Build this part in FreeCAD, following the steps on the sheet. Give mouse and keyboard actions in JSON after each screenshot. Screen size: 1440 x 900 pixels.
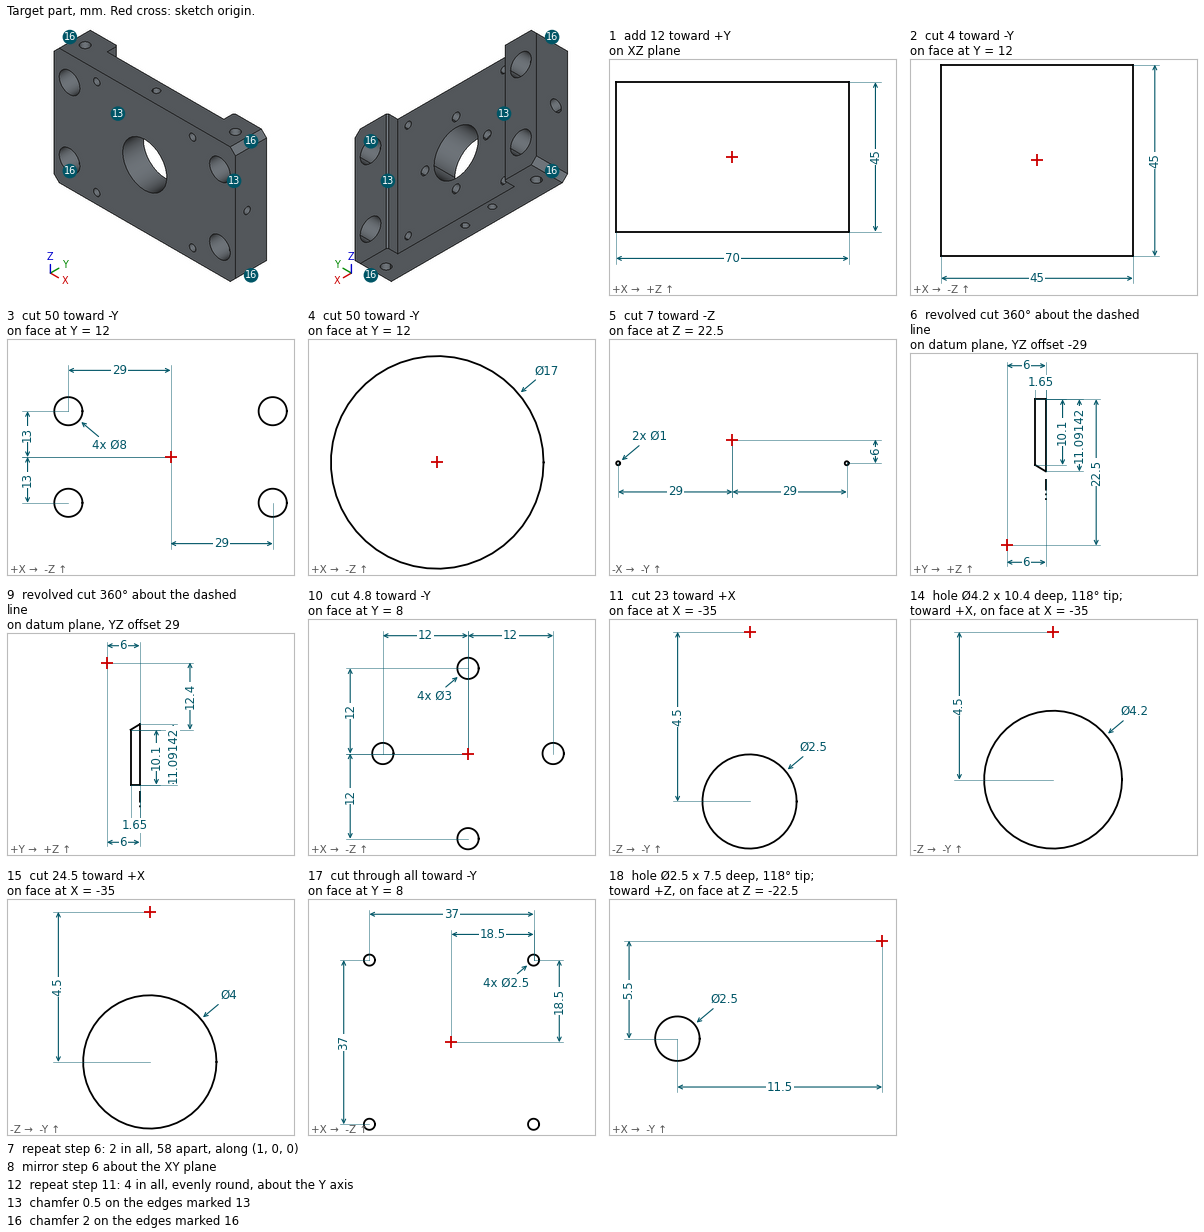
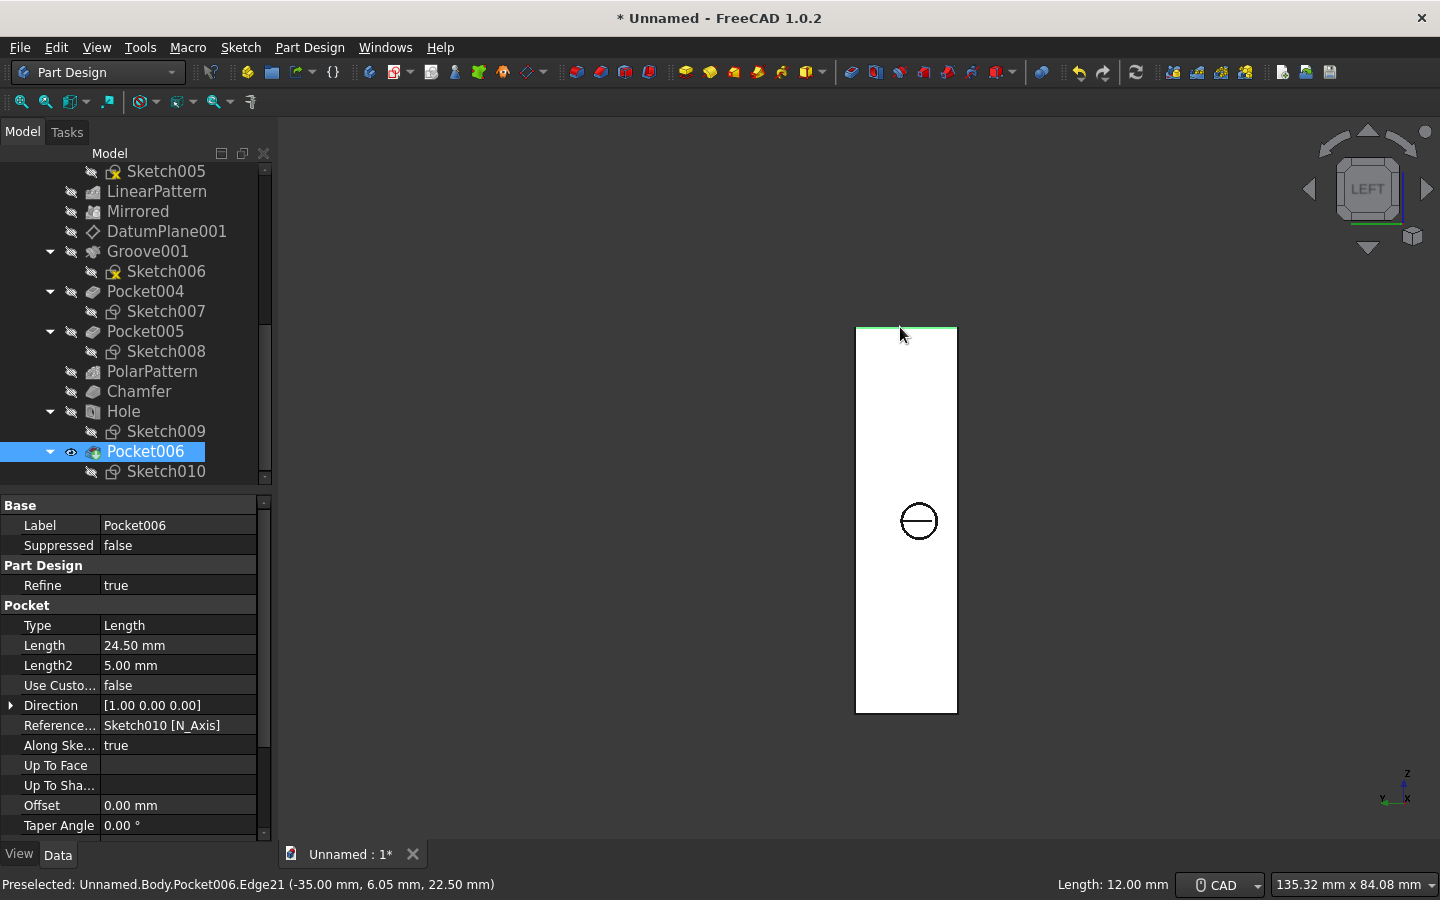
{"action": "left_click", "coordinate": [906, 713], "text": "ctrl"}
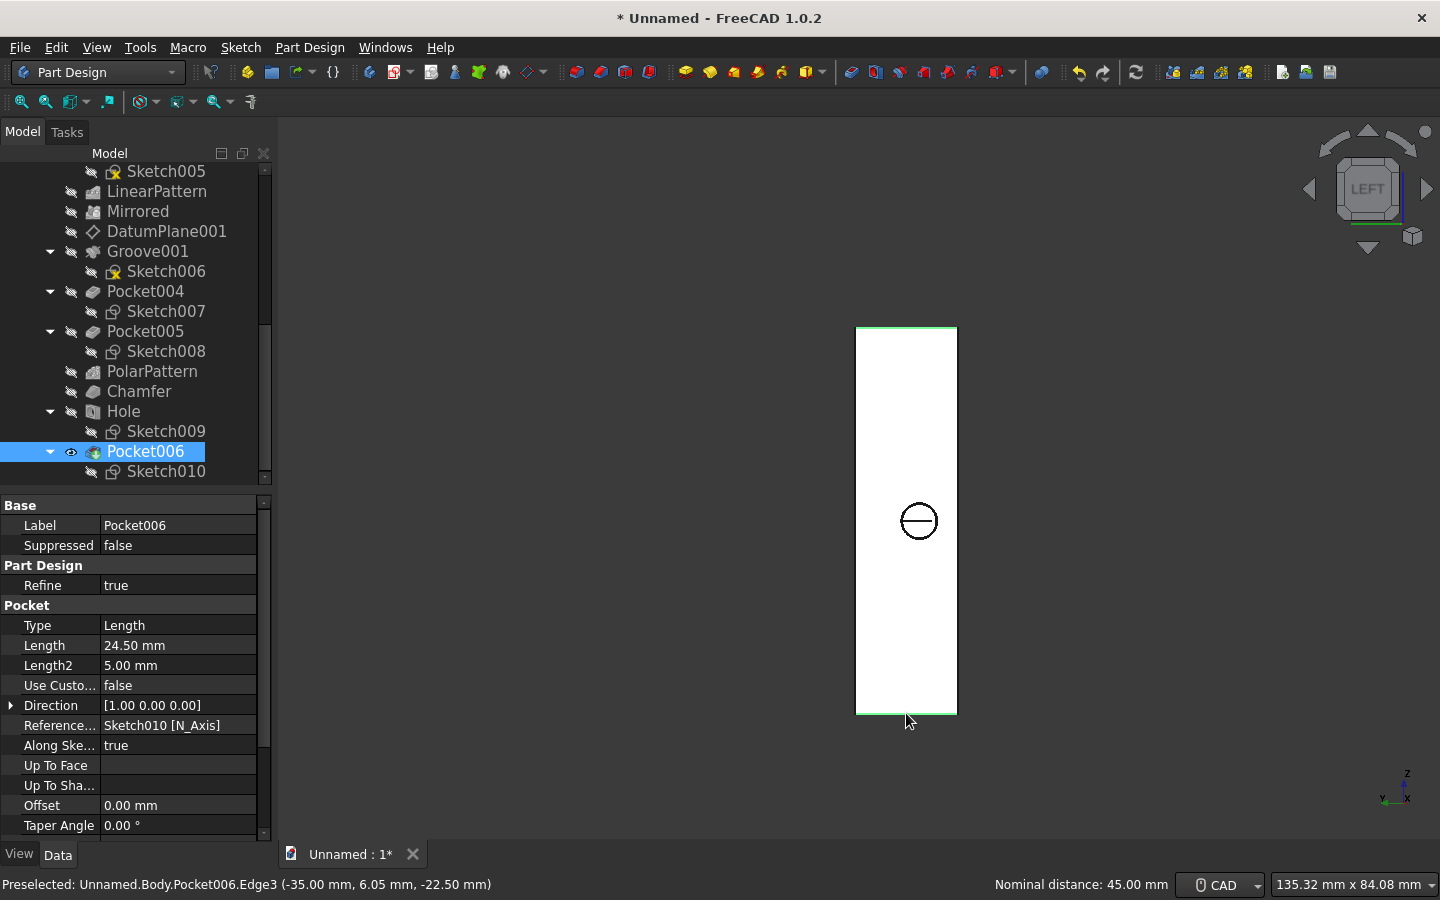
{"action": "key", "text": "0"}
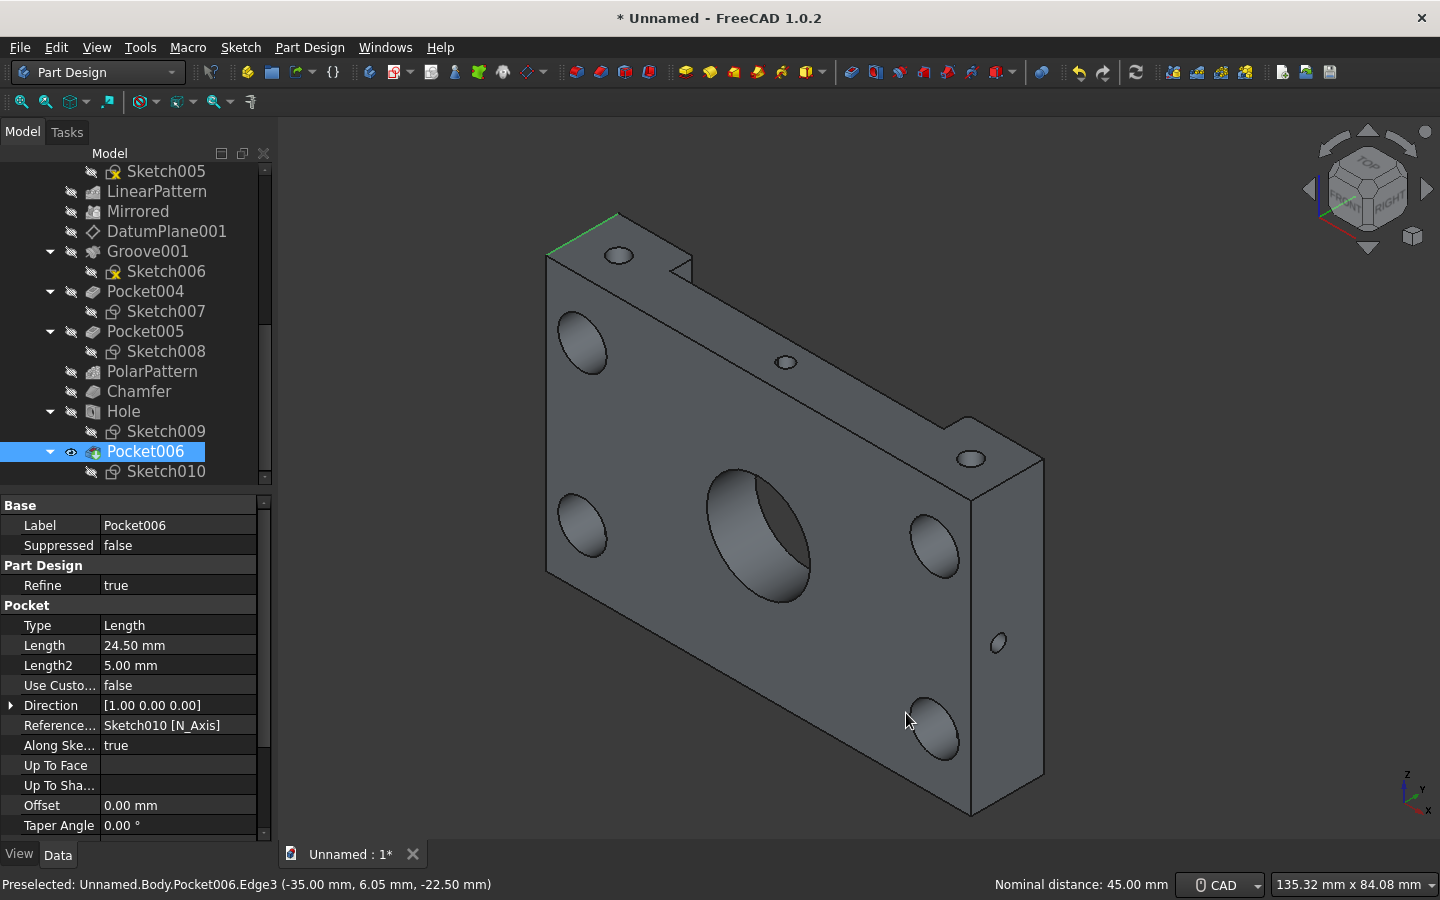
{"action": "left_click", "coordinate": [1007, 479], "text": "ctrl"}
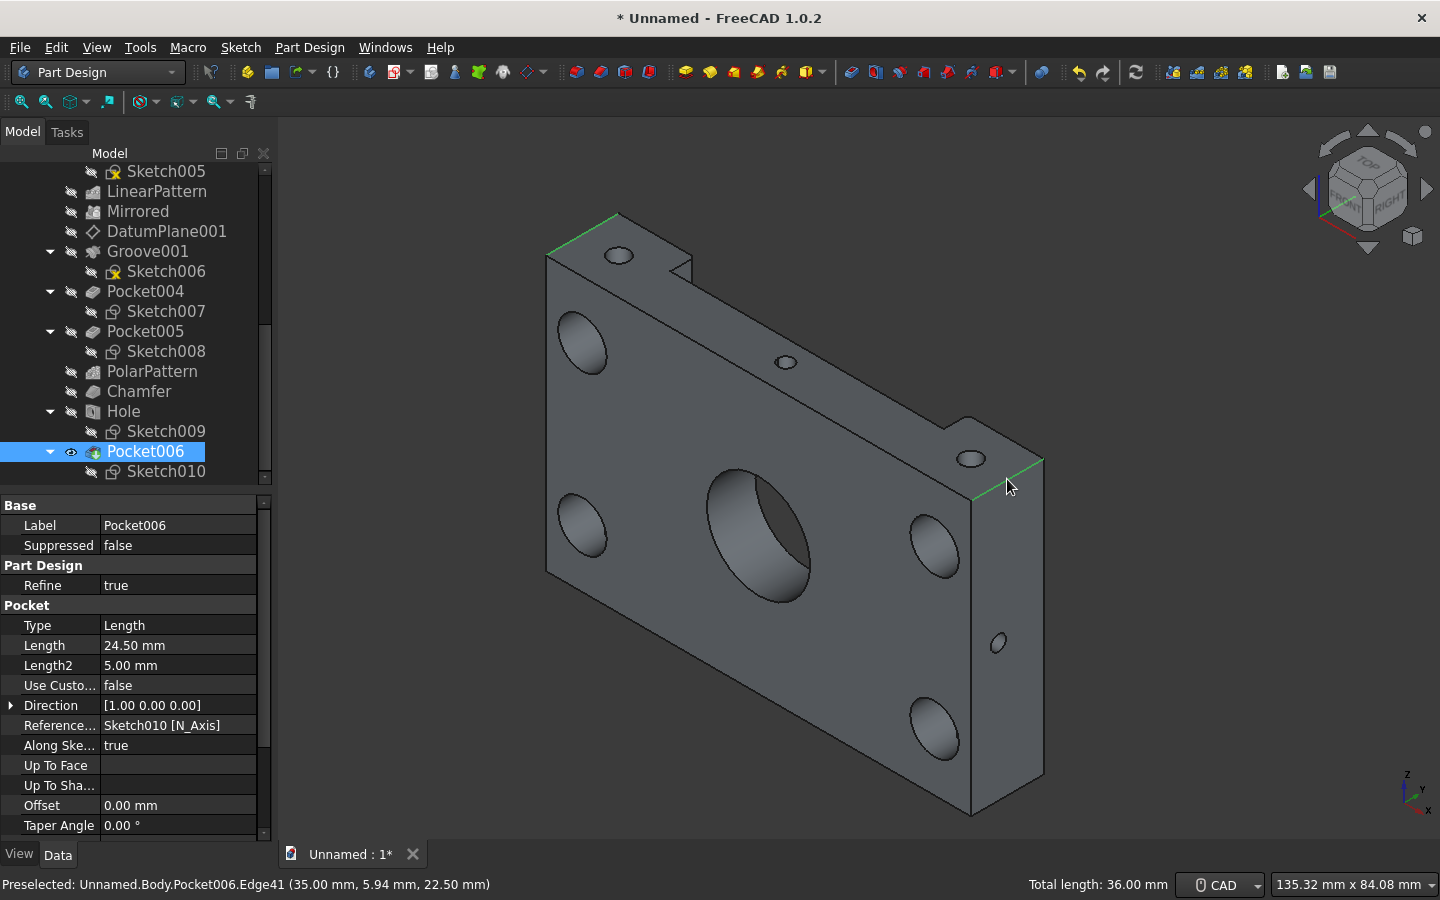
{"action": "key", "text": "2"}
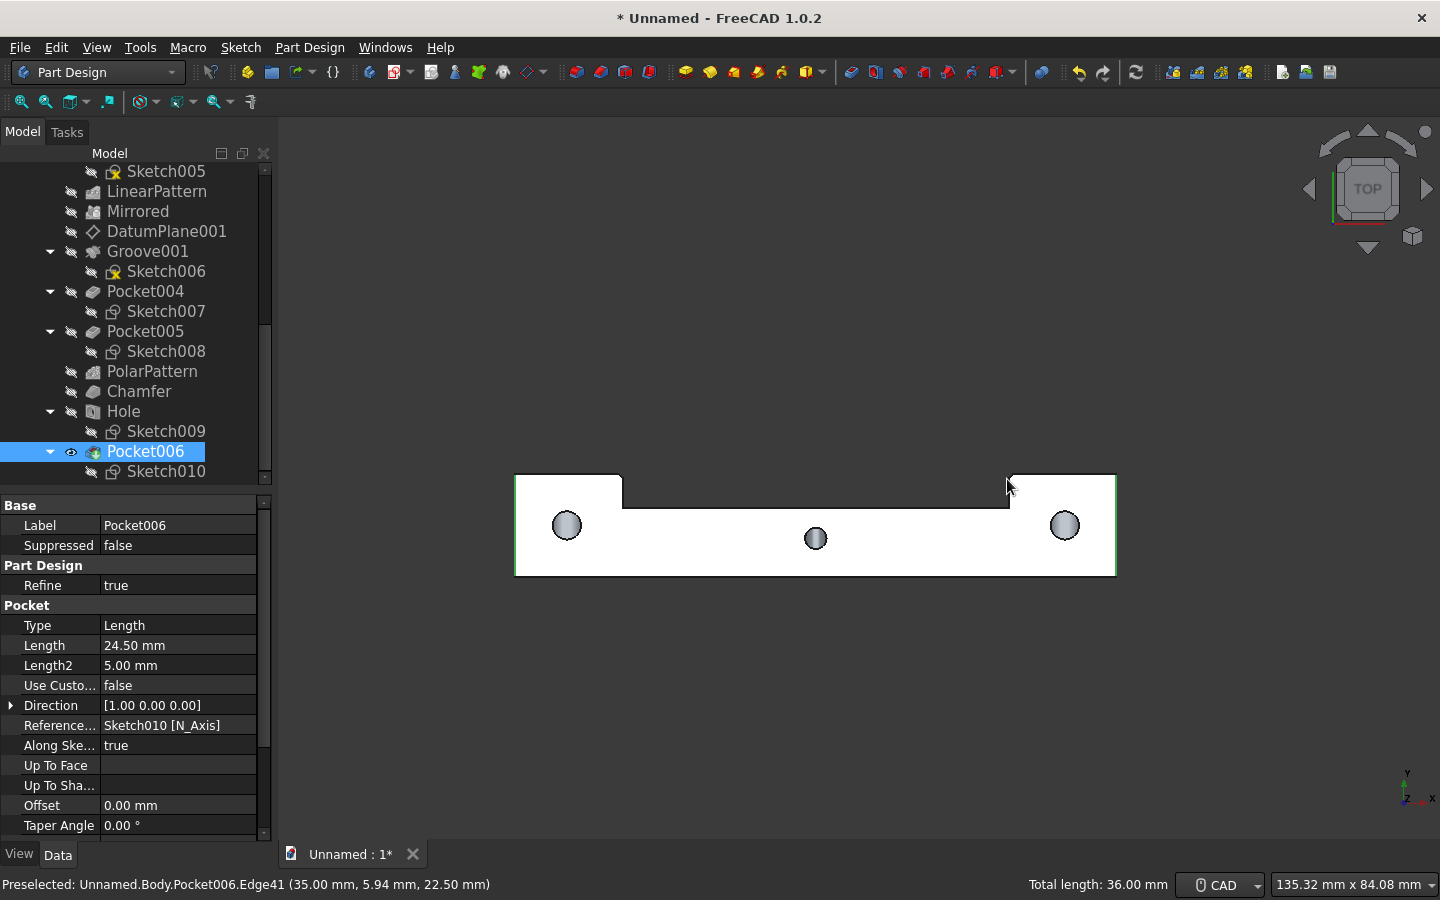
{"action": "key", "text": "1"}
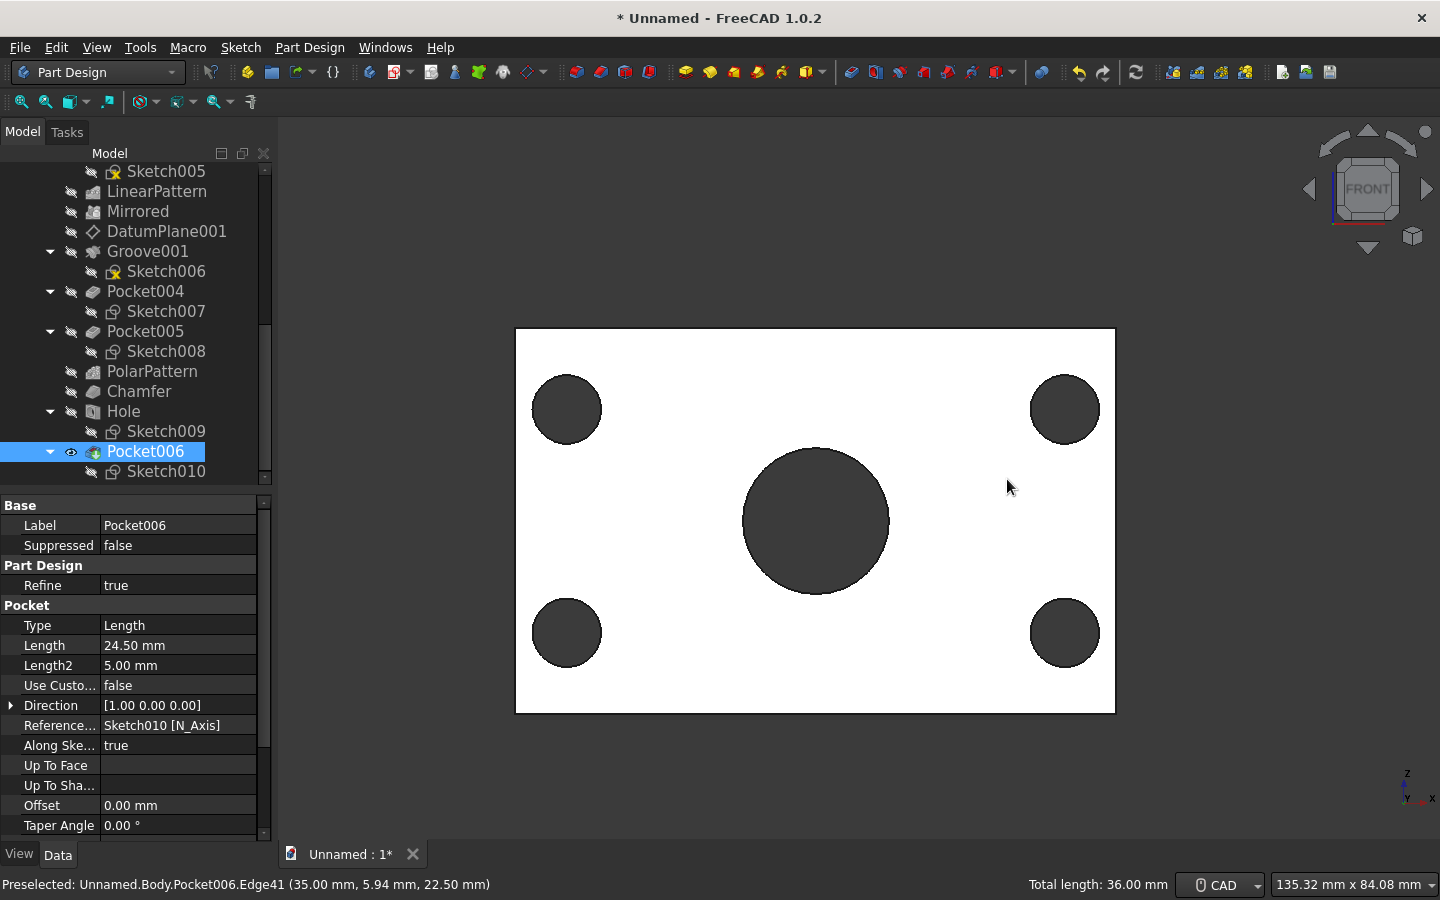
{"action": "key", "text": "3"}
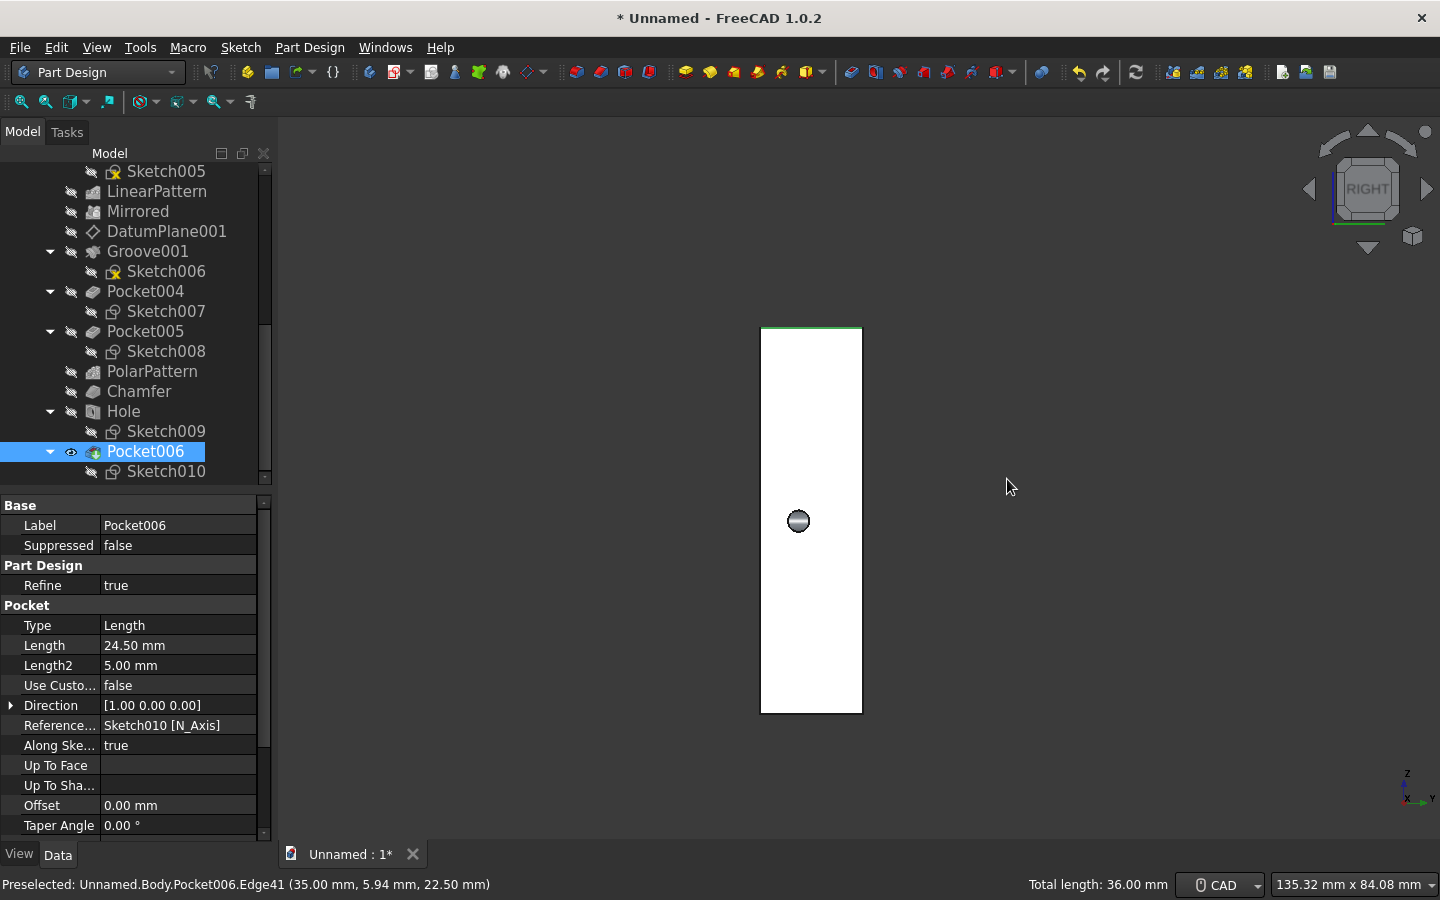
{"action": "left_click", "coordinate": [812, 713], "text": "ctrl"}